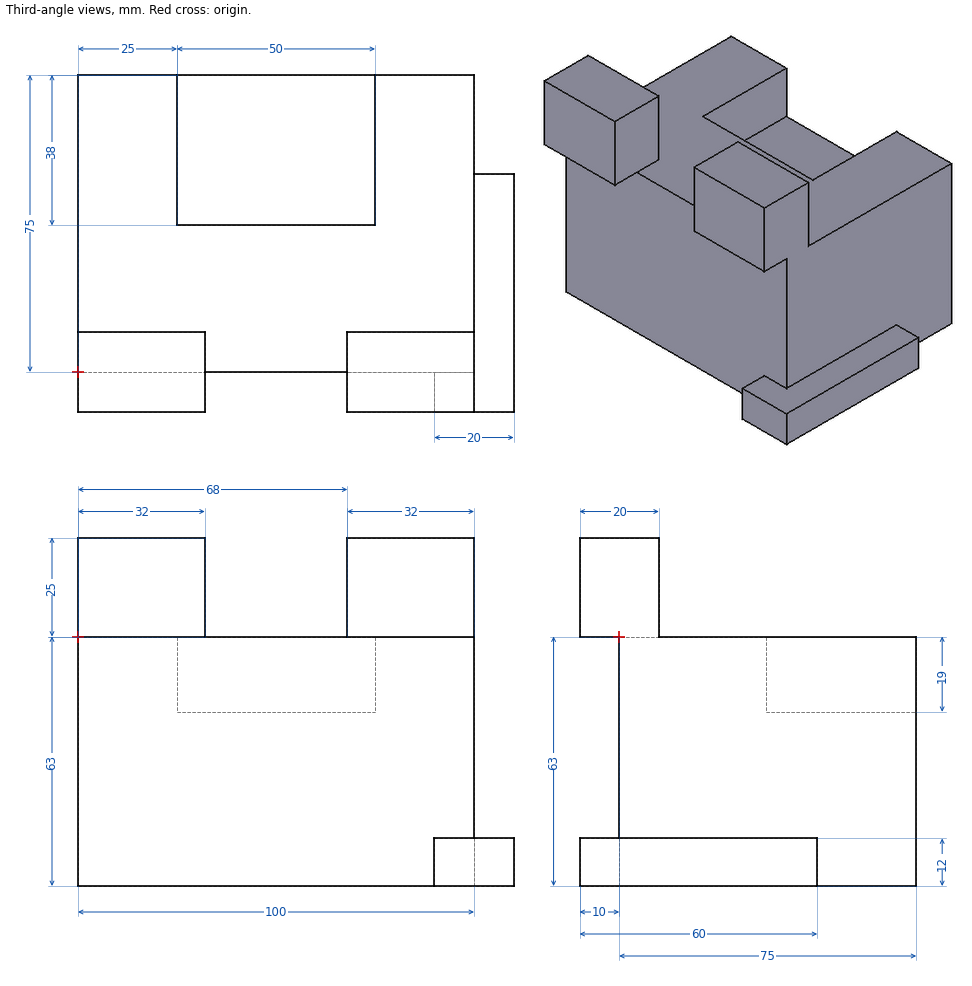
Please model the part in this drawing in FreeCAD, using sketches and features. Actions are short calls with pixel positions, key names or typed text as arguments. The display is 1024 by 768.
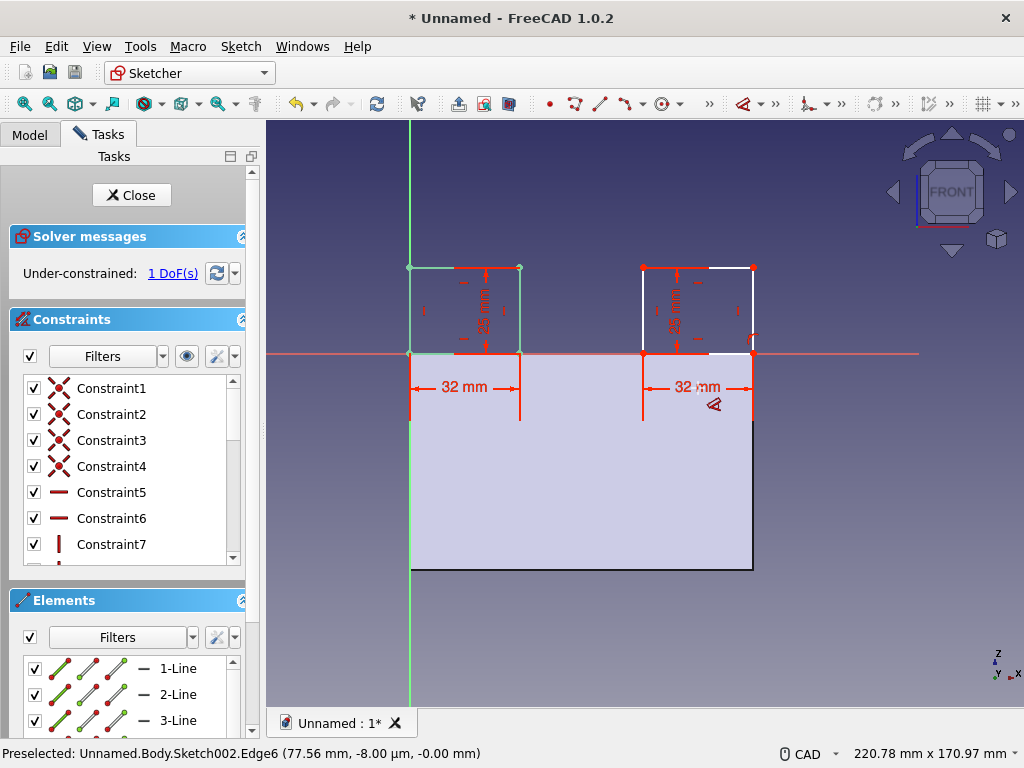
click(643, 268)
click(580, 388)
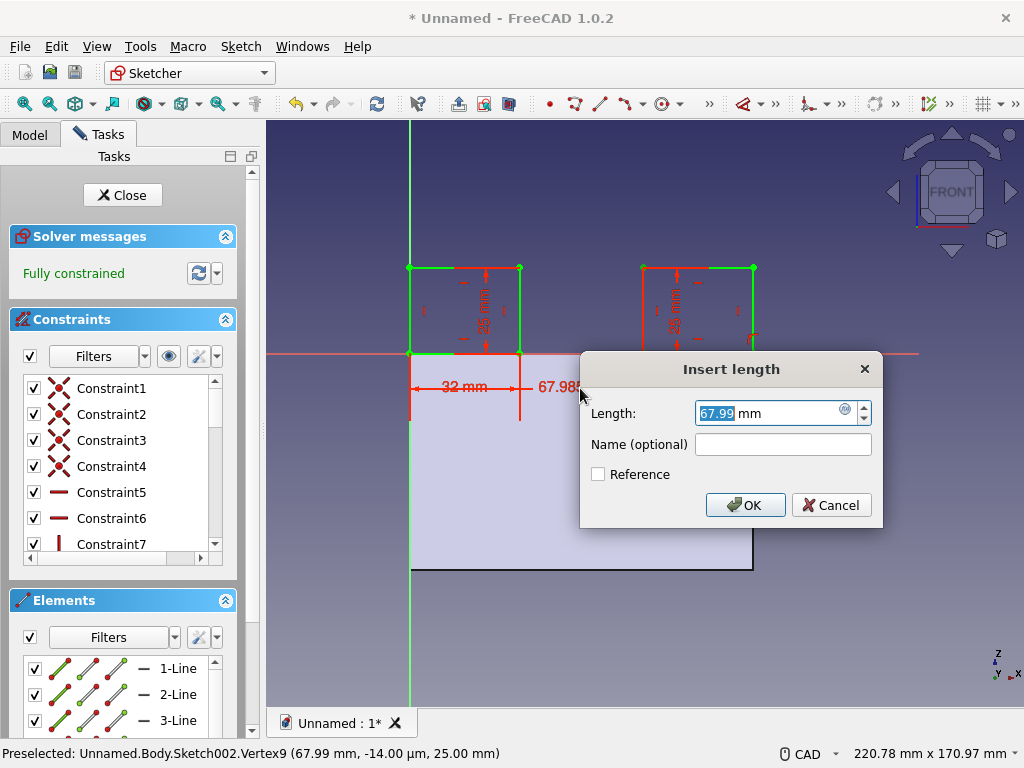
text(68)
key(Return)
key(Escape)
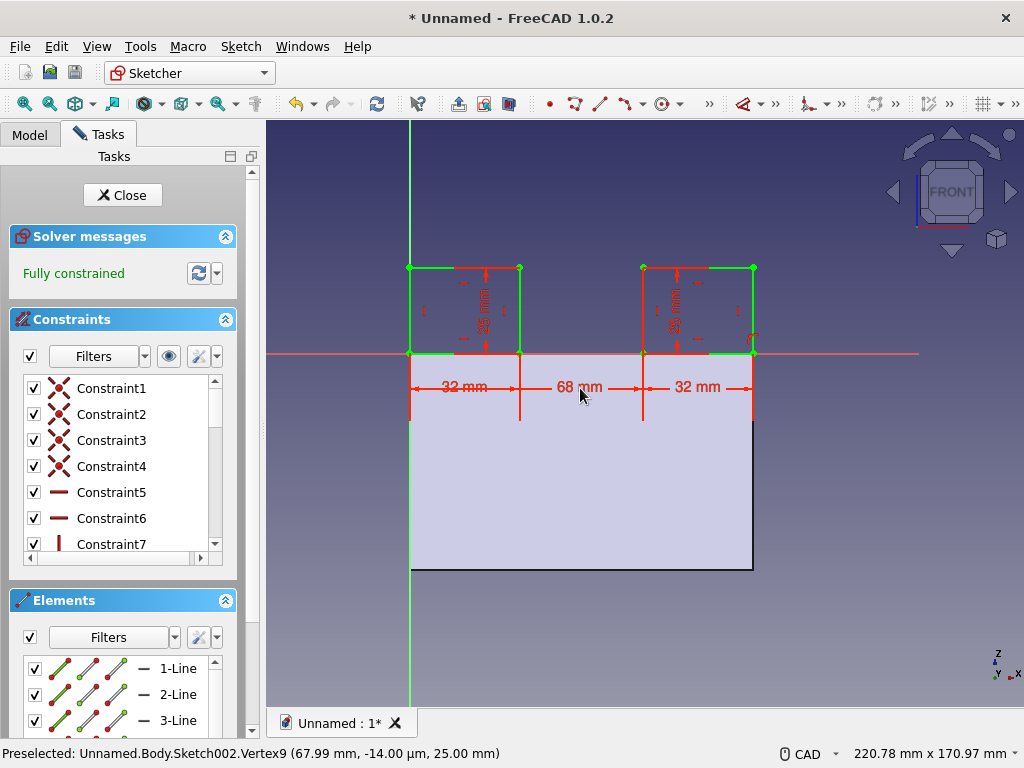
click(123, 195)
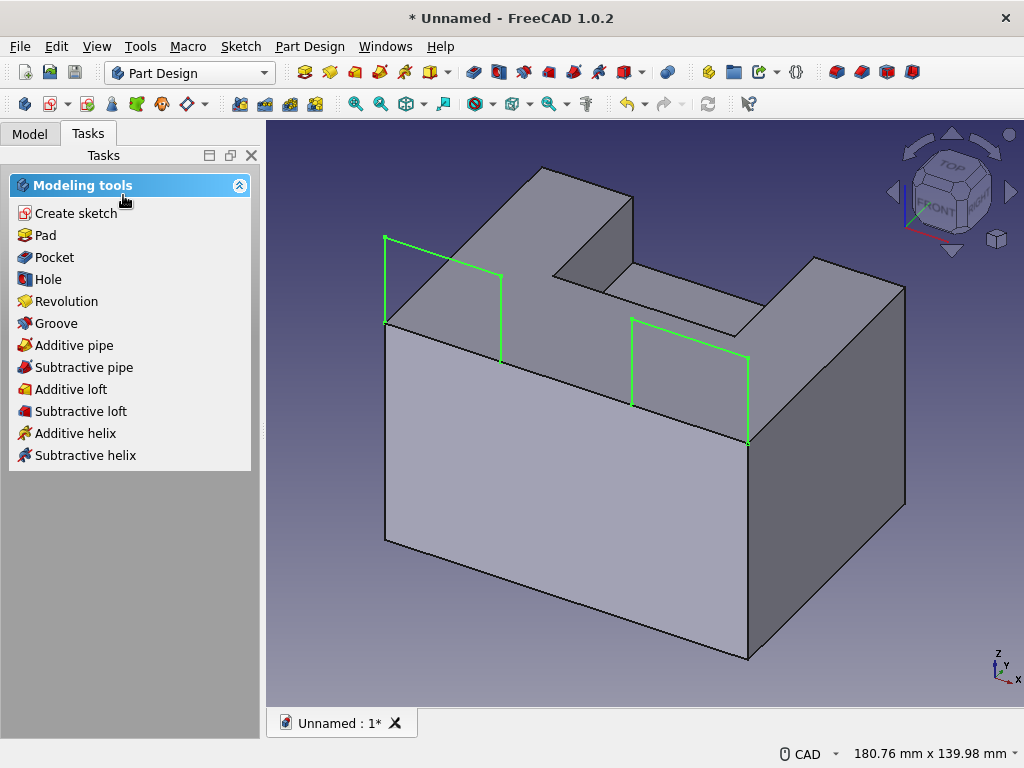
click(305, 72)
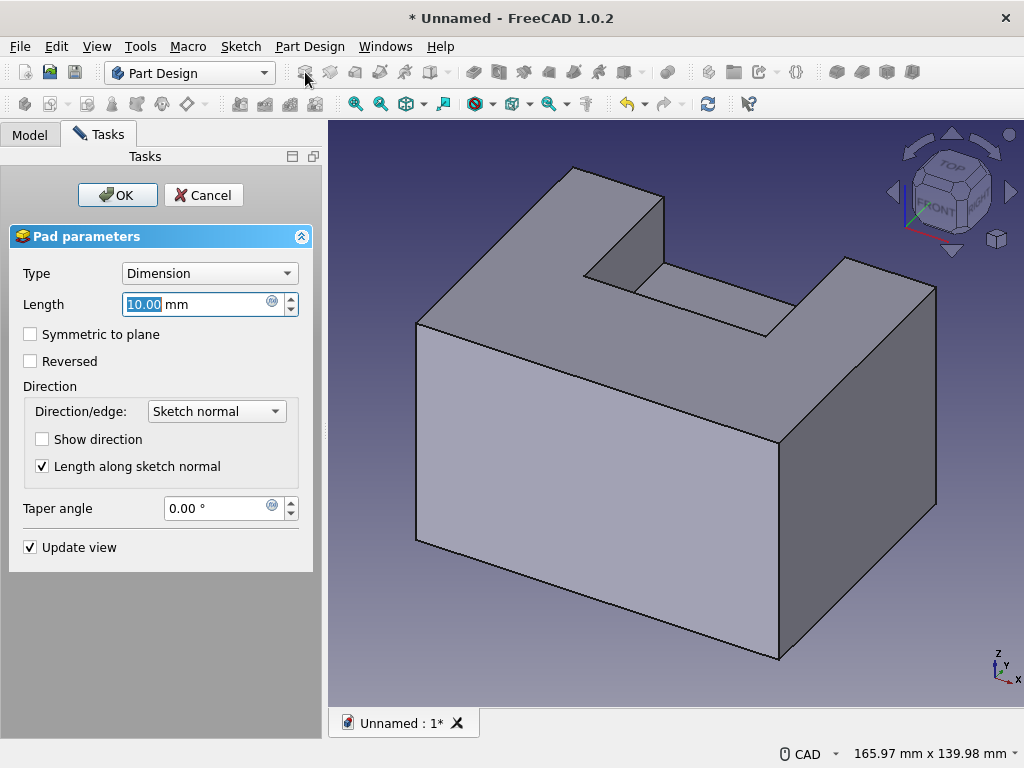
text(20)
key(Tab)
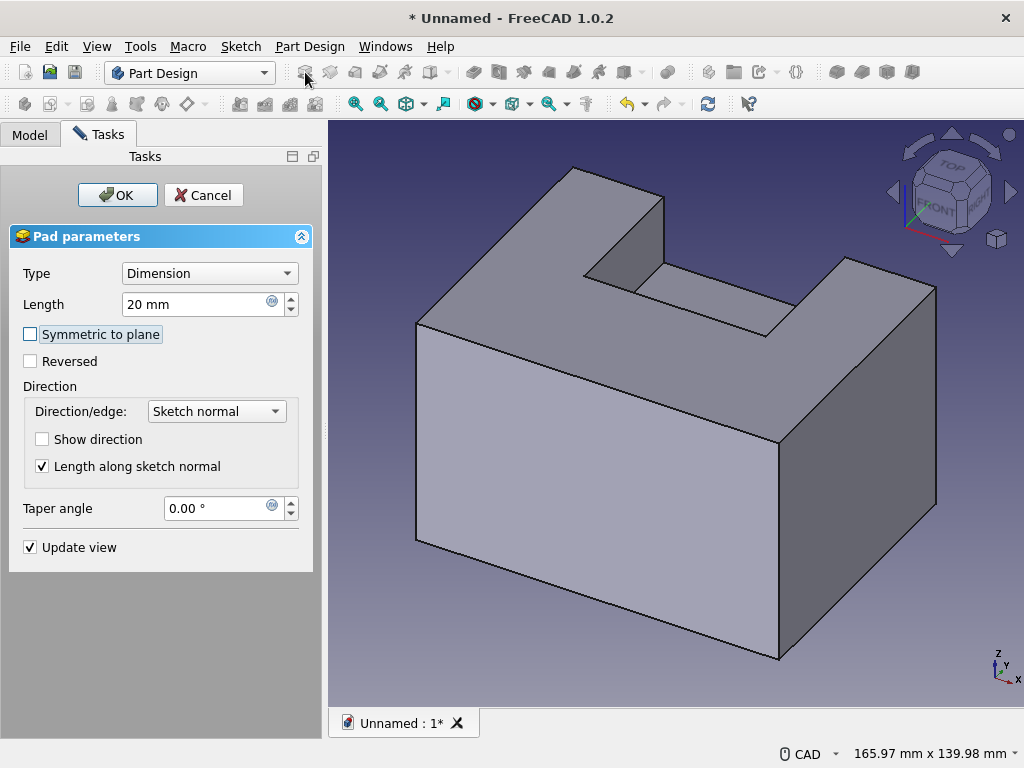
click(31, 334)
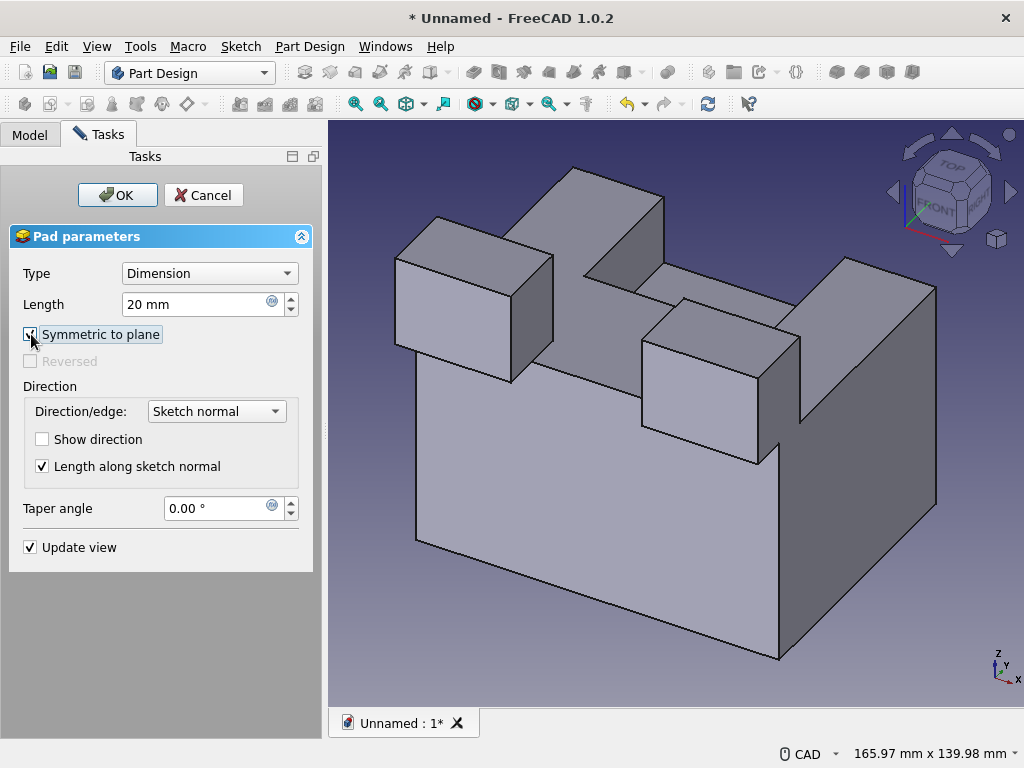
click(118, 195)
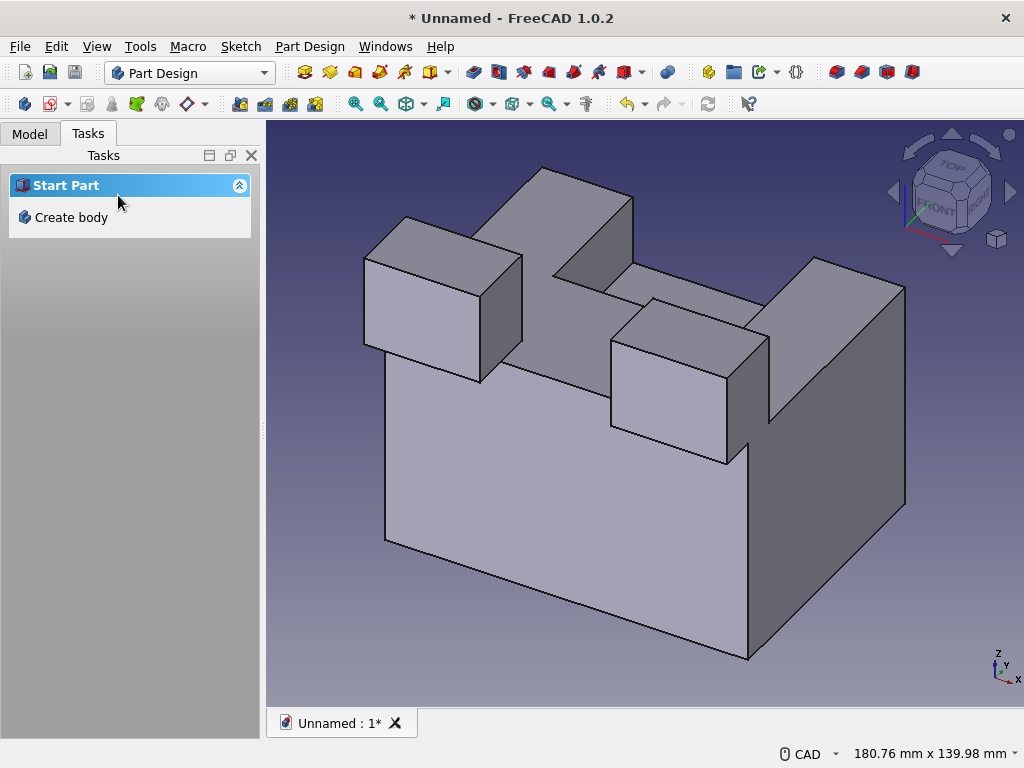
click(356, 104)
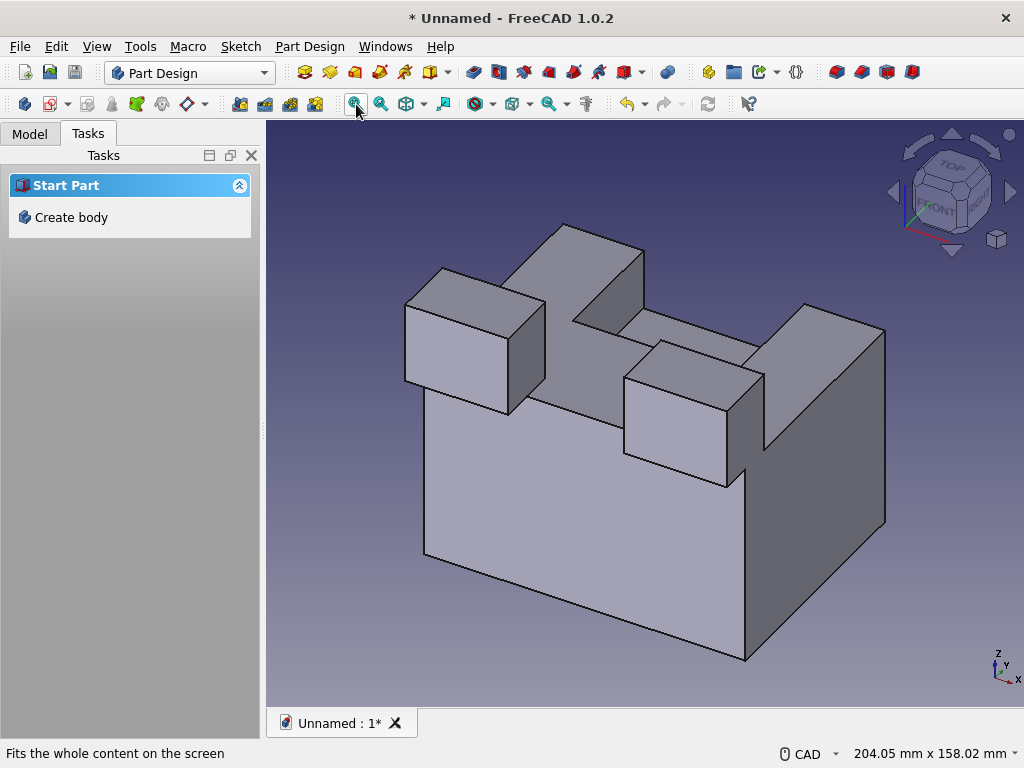
click(806, 504)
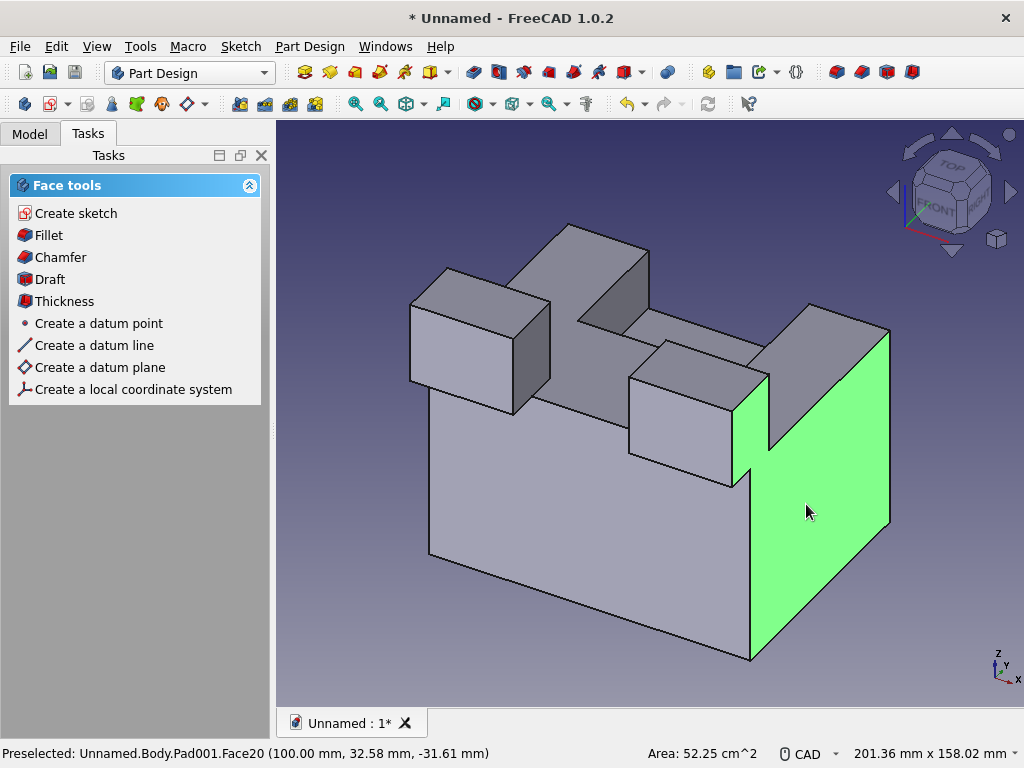
click(50, 104)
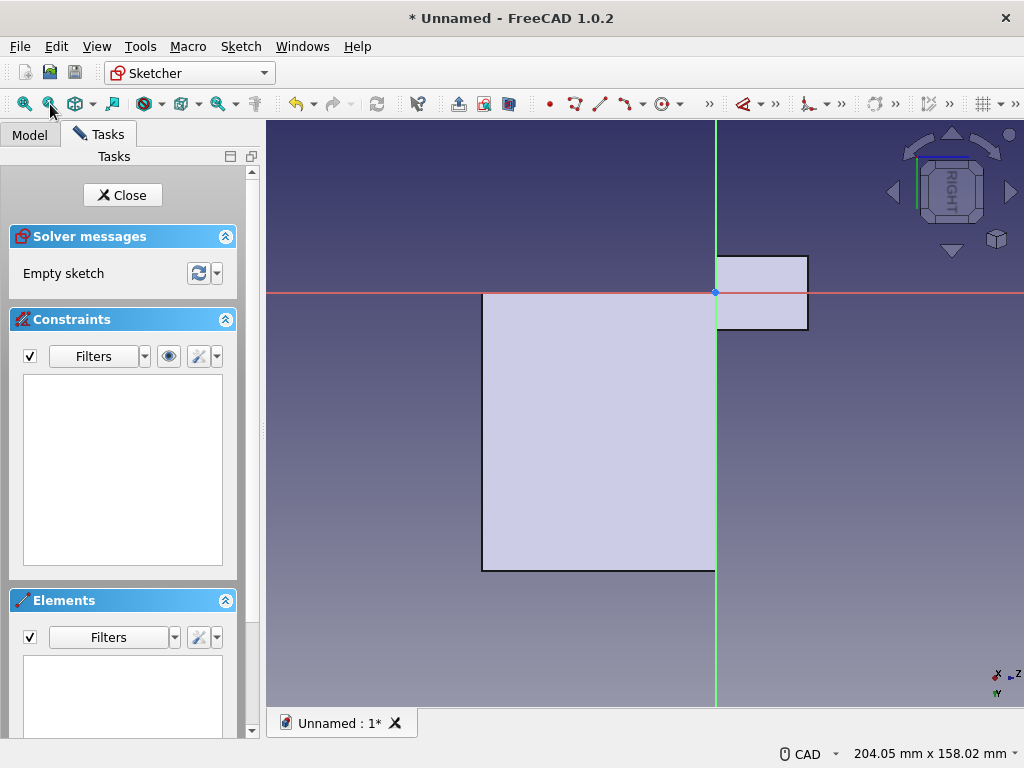
scroll(625, 311, up, 3)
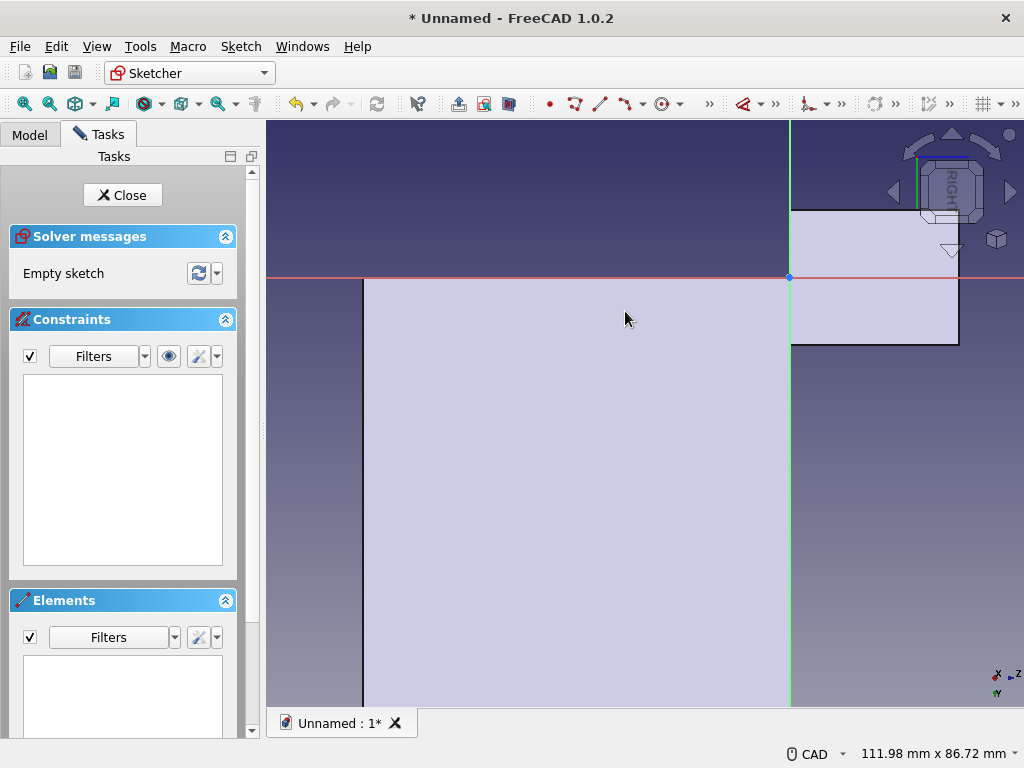
key(g)
key(r)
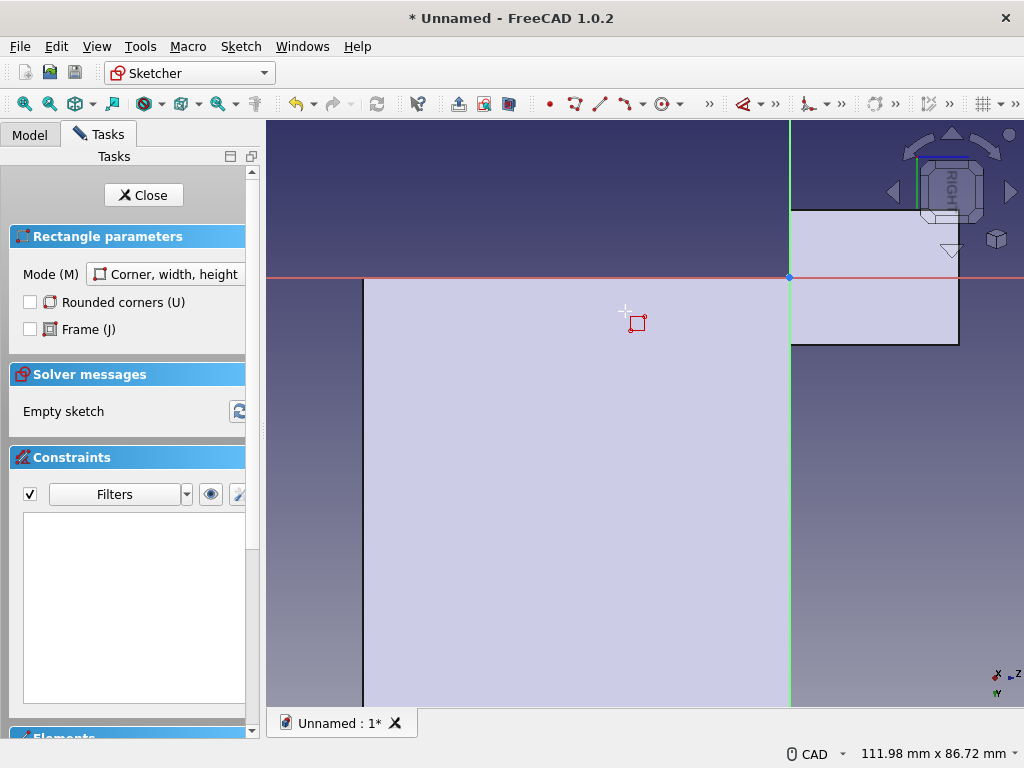
click(363, 210)
click(444, 616)
key(Escape)